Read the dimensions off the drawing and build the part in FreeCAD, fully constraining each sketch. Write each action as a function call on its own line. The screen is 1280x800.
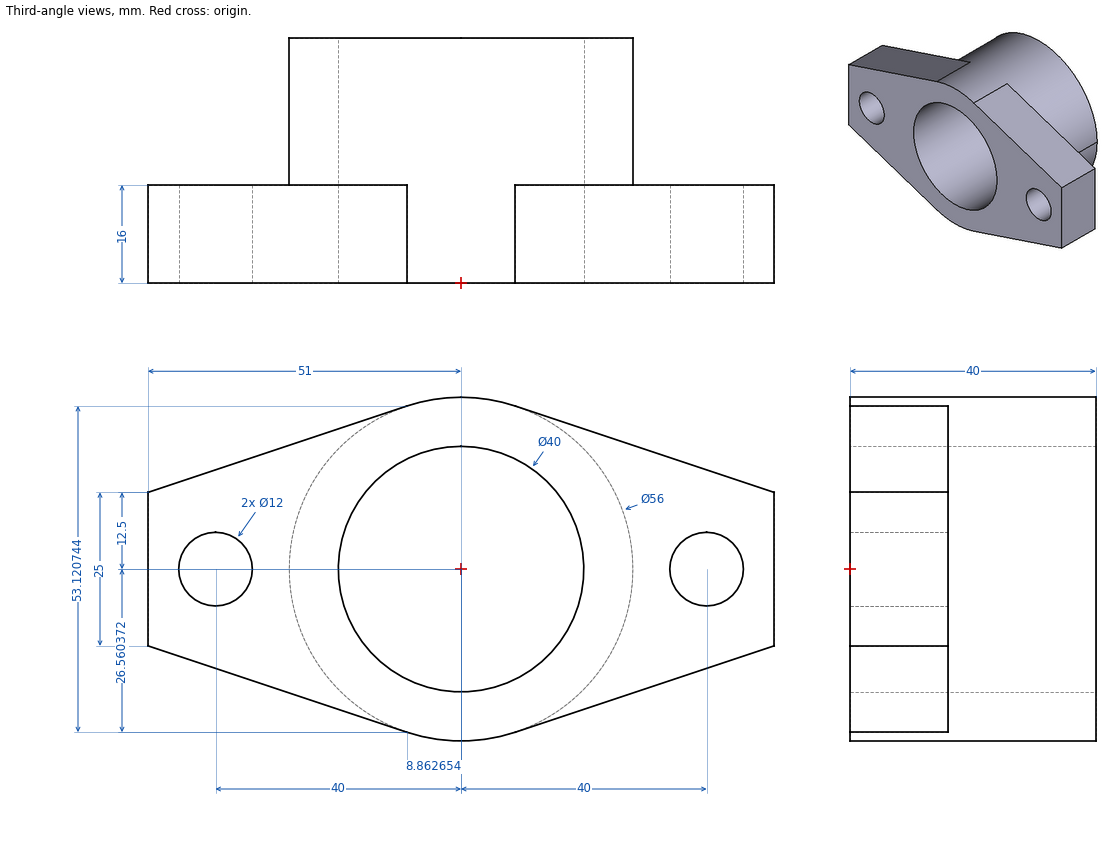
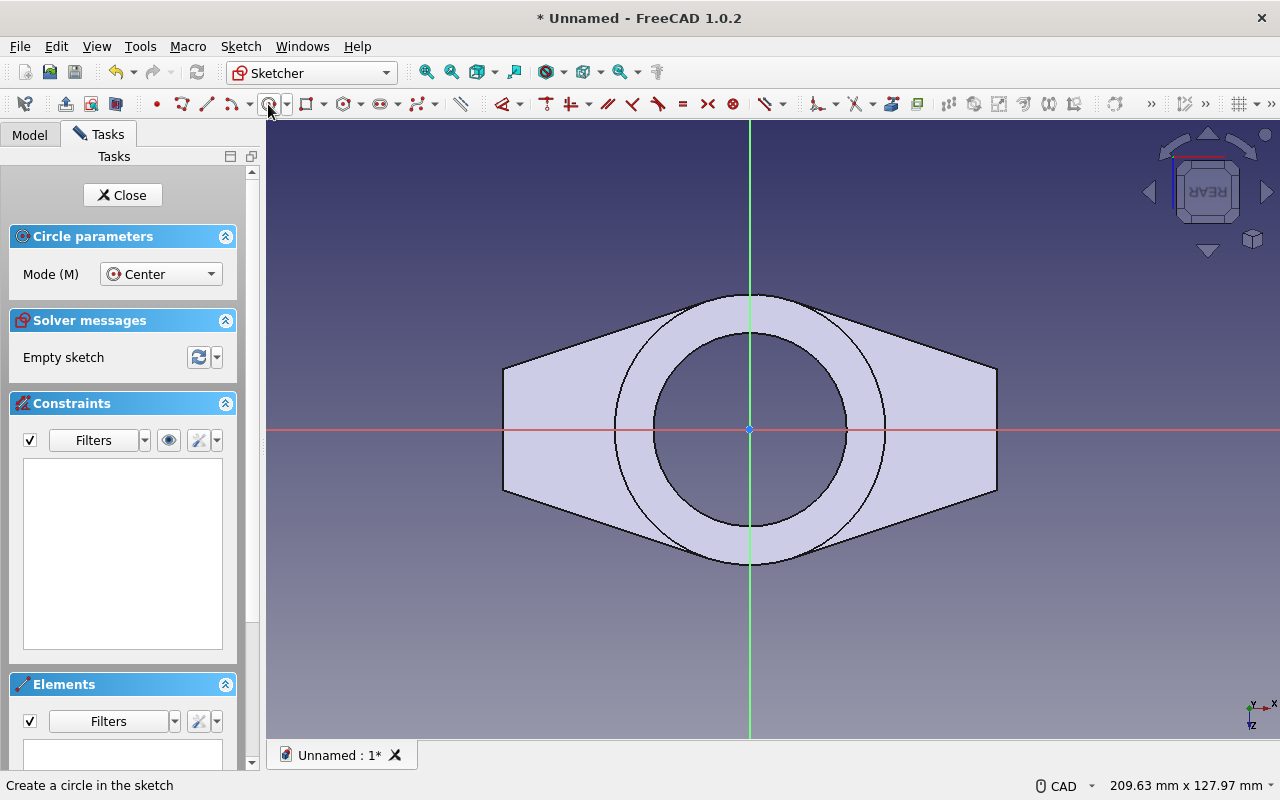
click(557, 430)
move(577, 409)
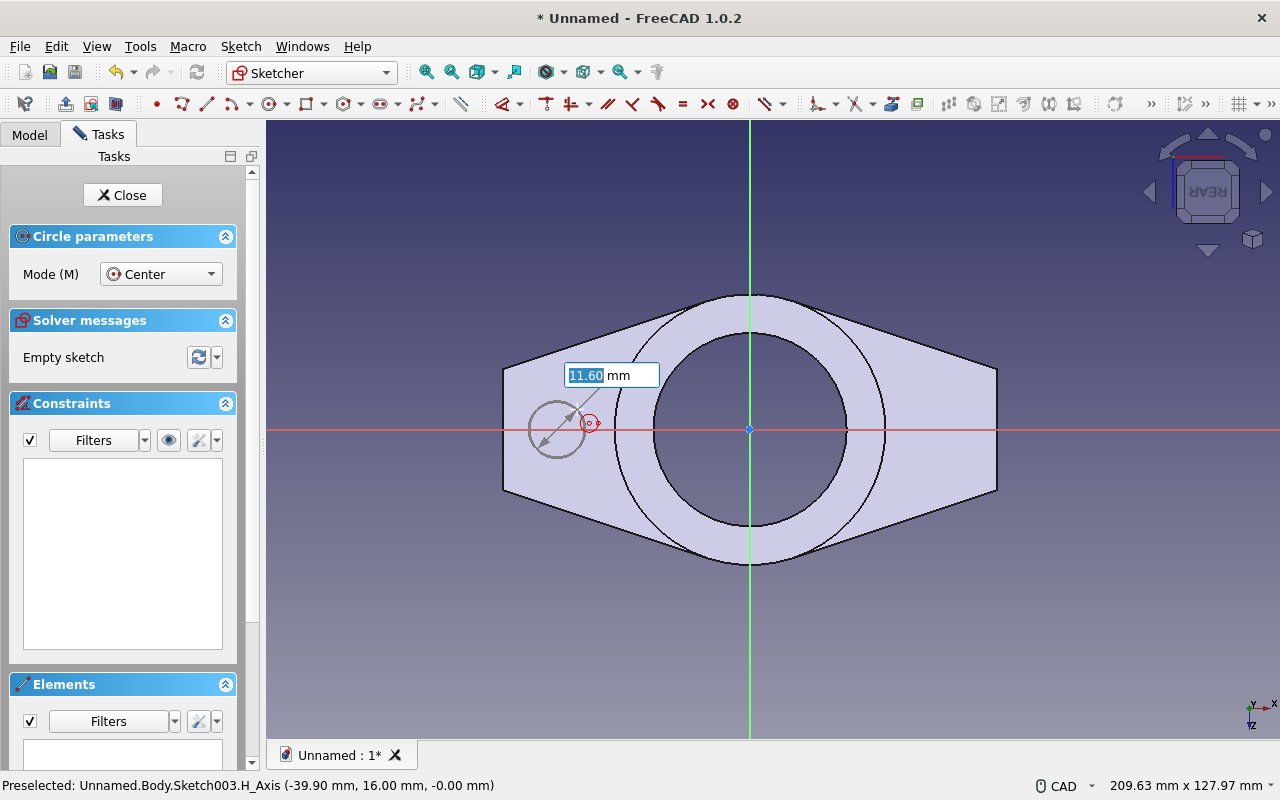
text(12)
key(Return)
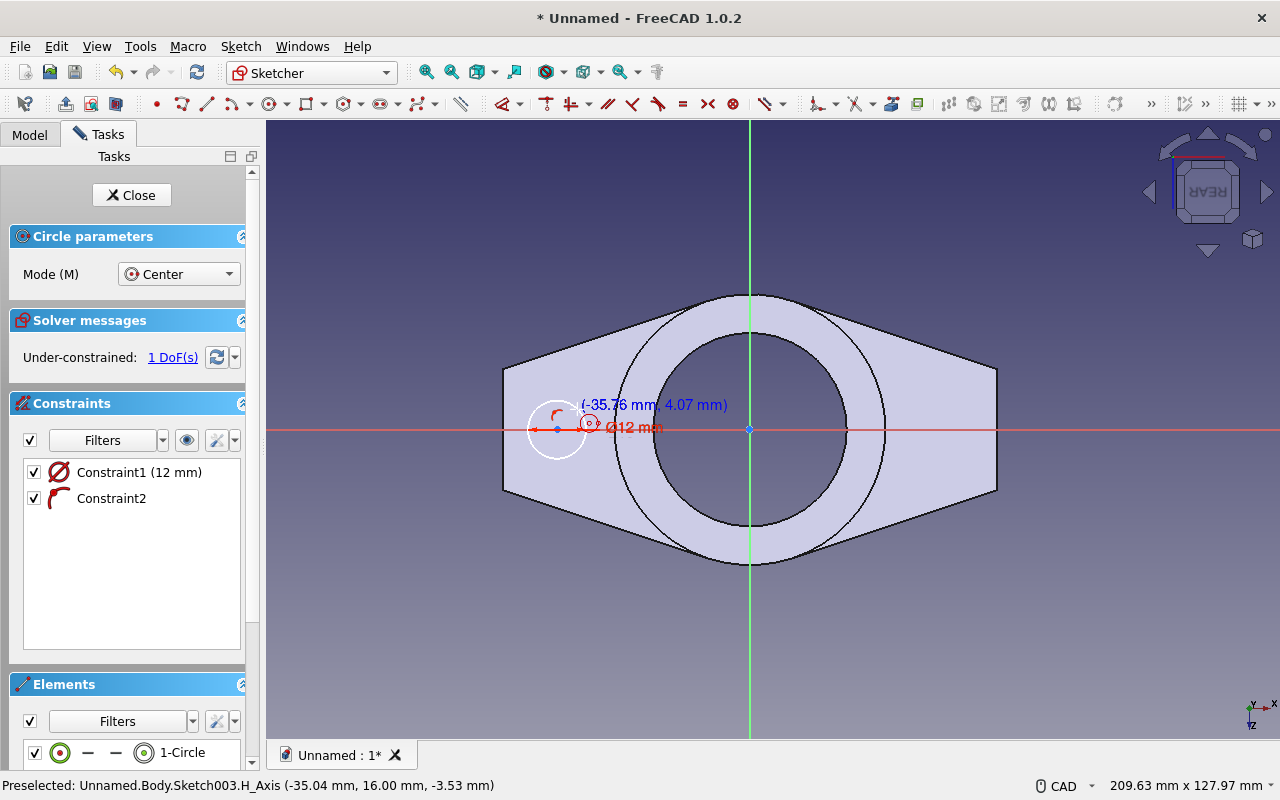
click(943, 430)
move(964, 409)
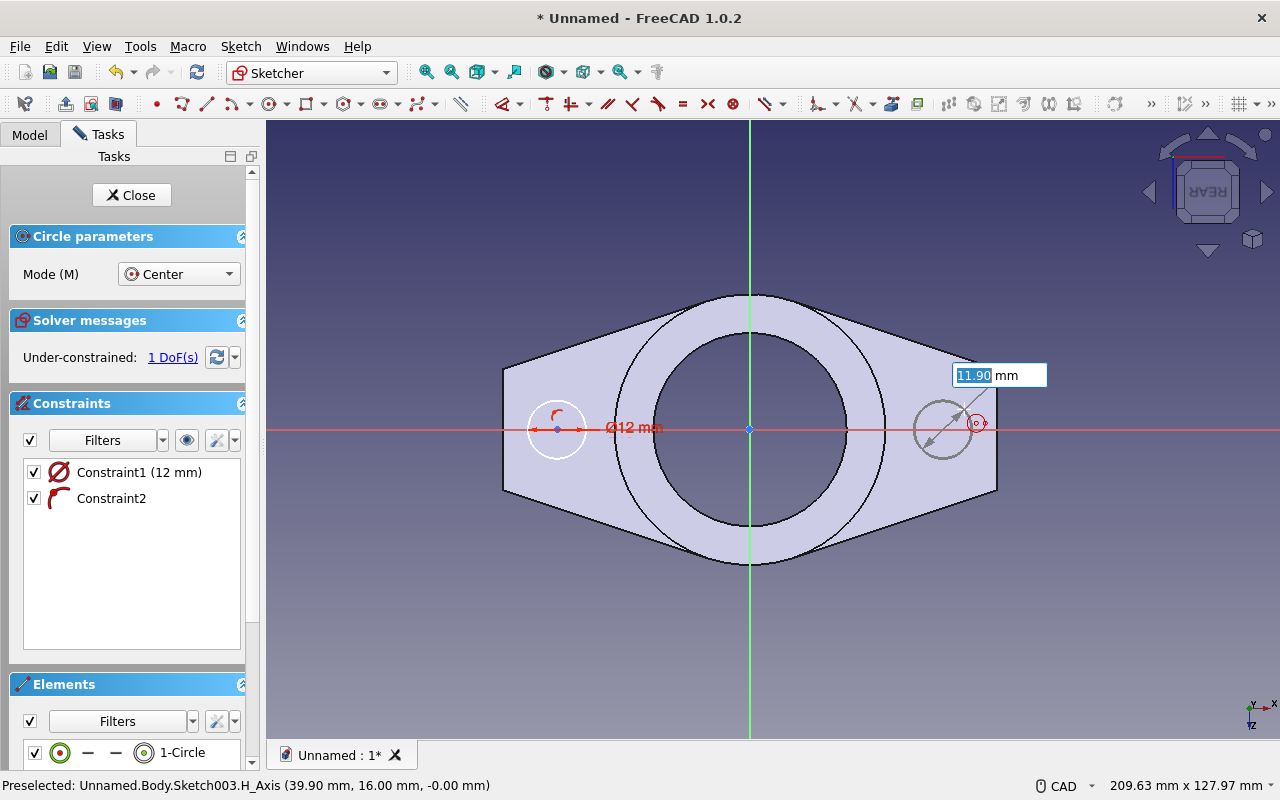
text(12)
key(Return)
key(Escape)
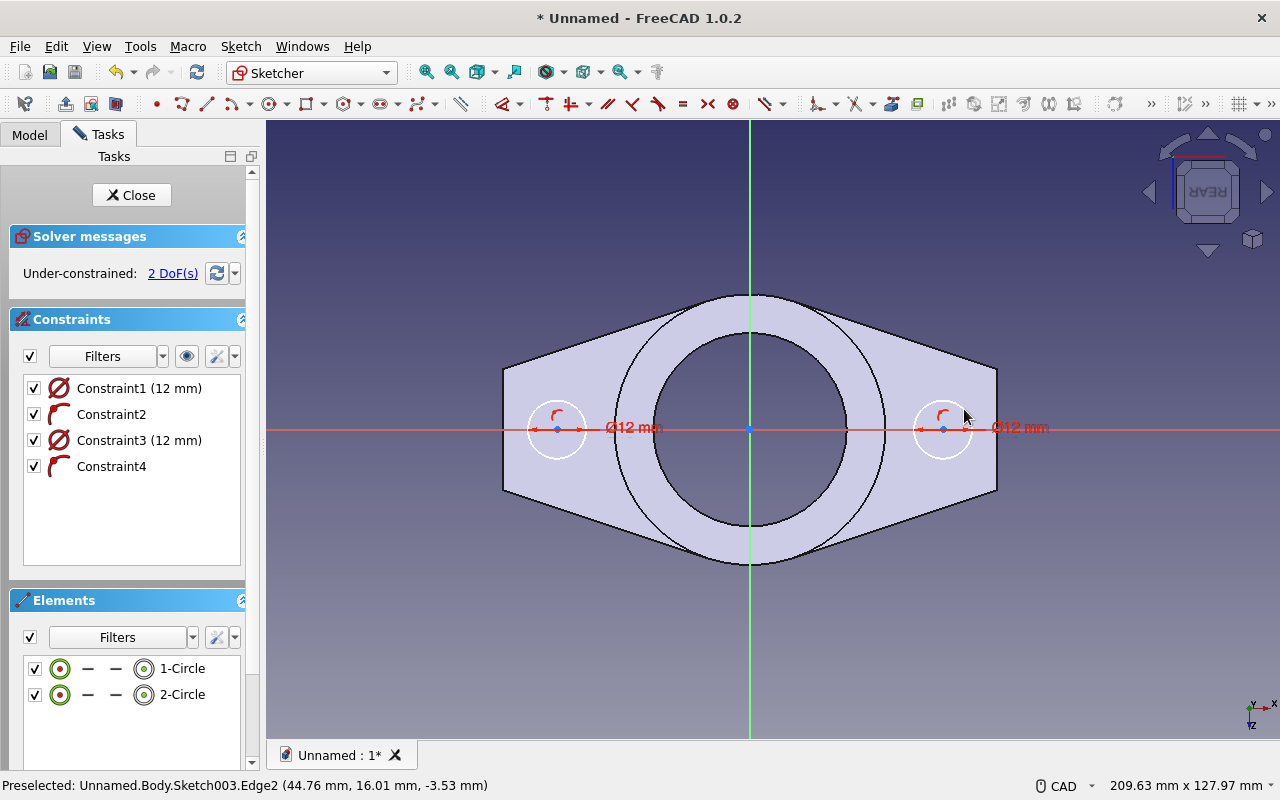
click(502, 104)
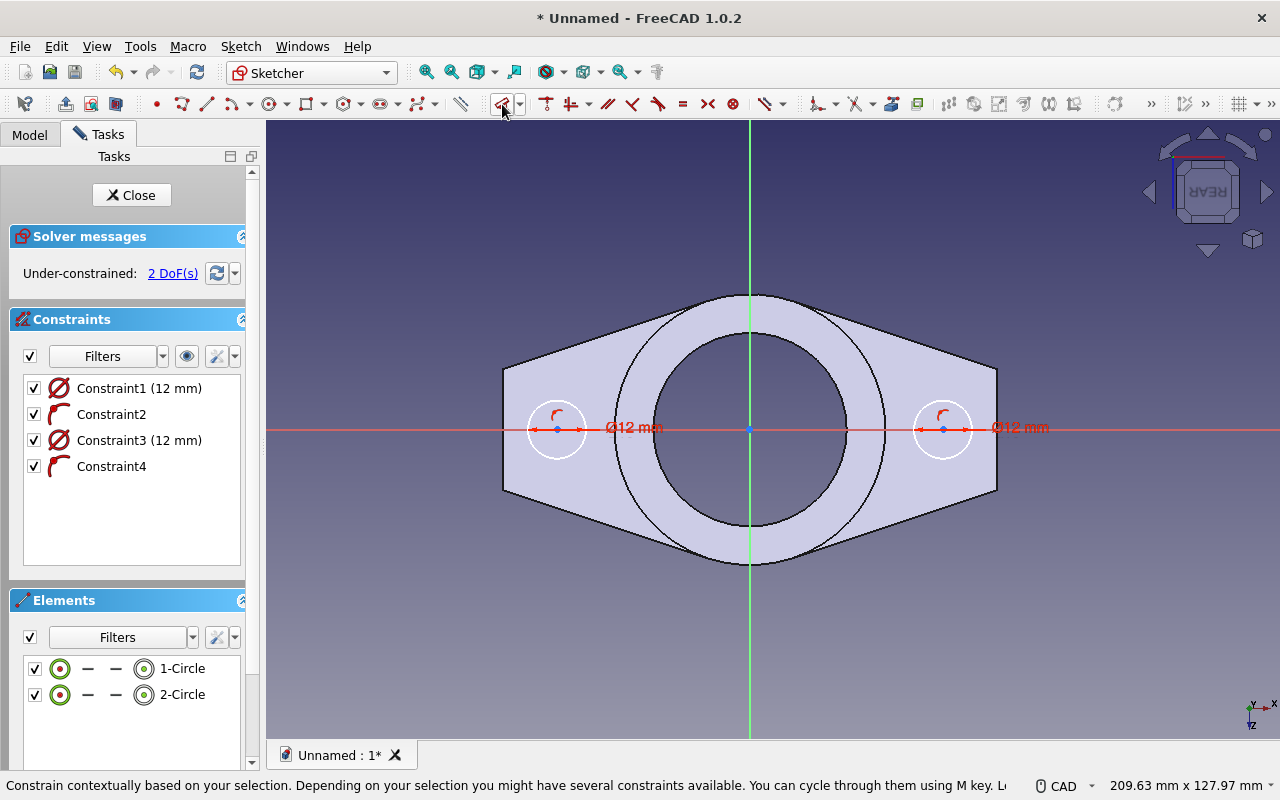
click(557, 430)
click(653, 464)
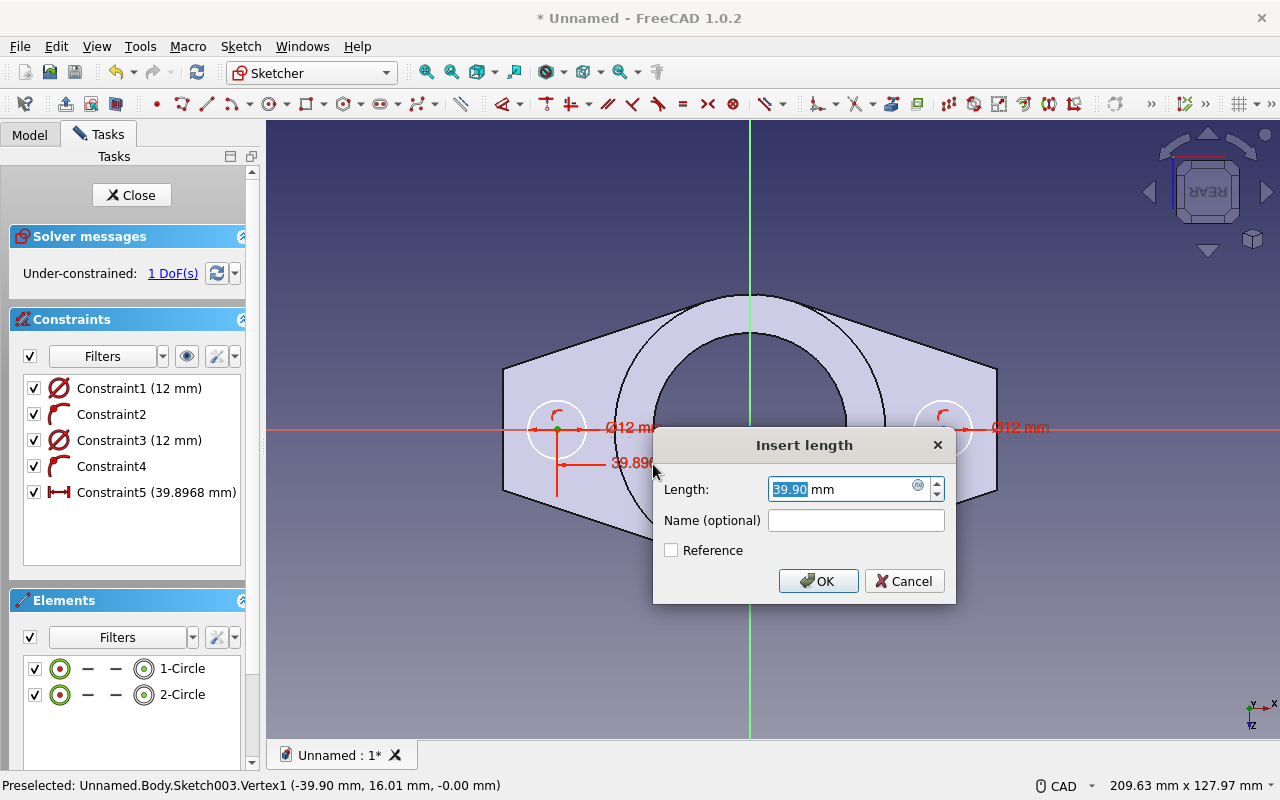
text(40)
key(Return)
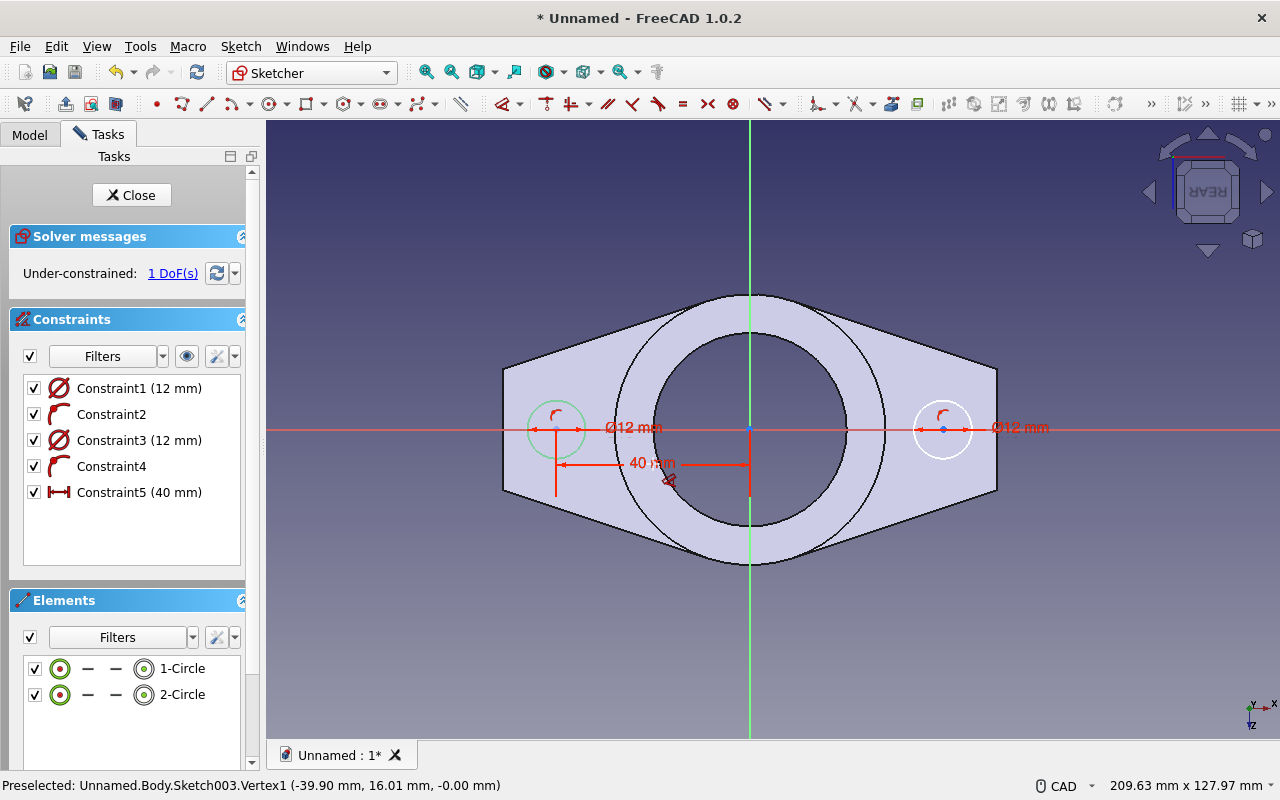
click(943, 430)
click(846, 464)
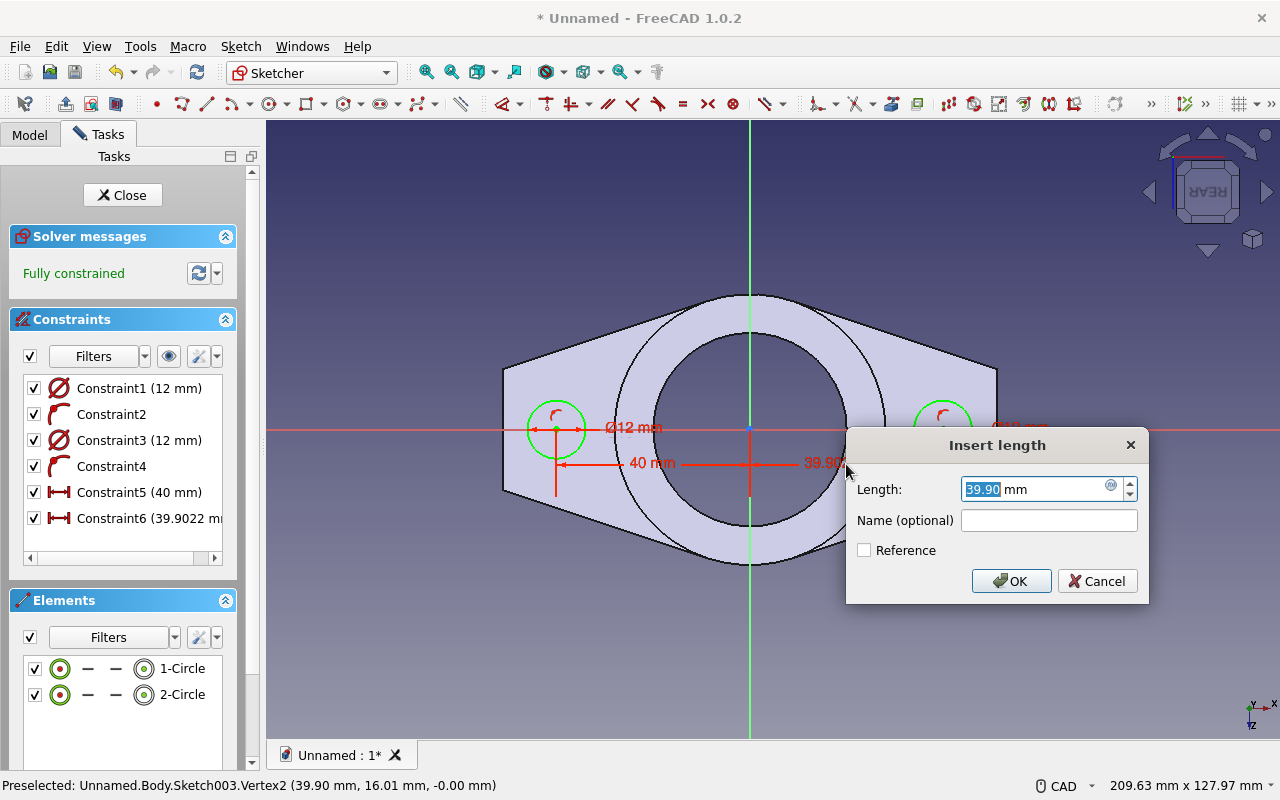
text(40)
key(Return)
key(Escape)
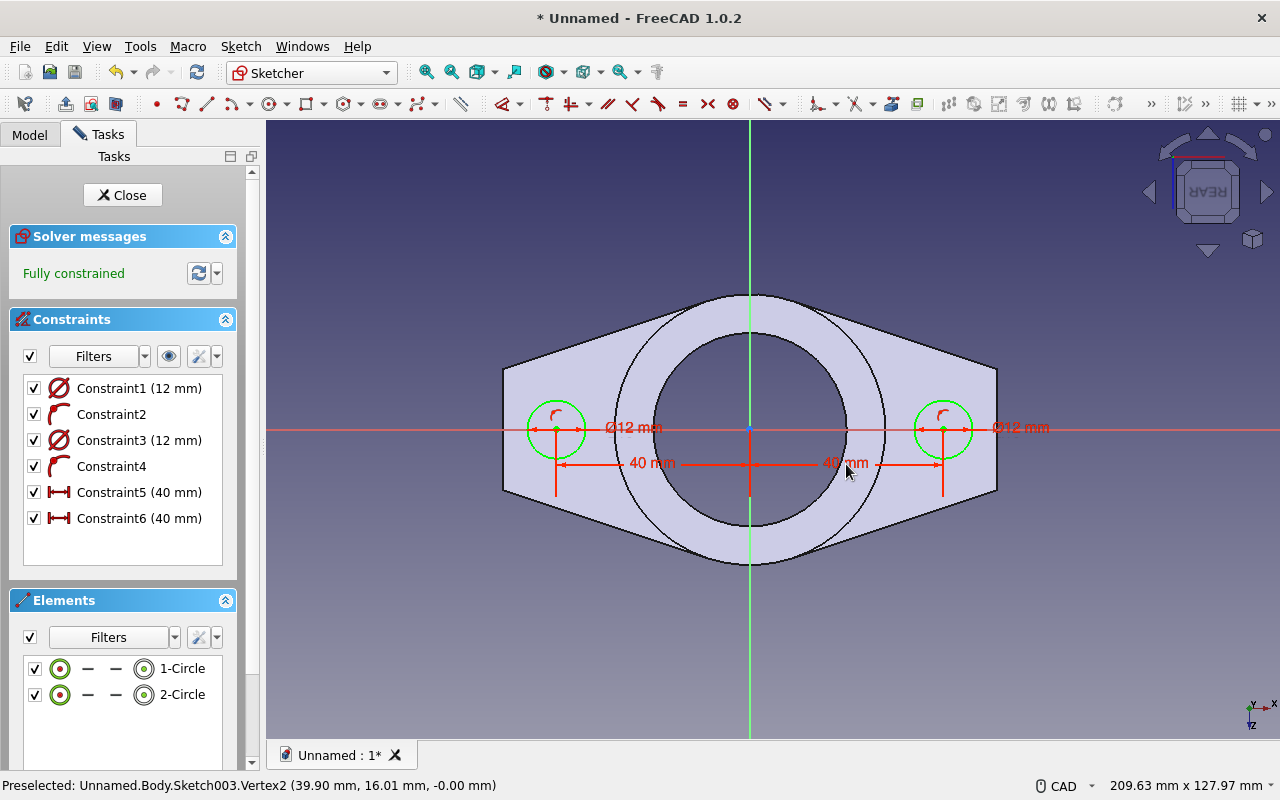
click(123, 195)